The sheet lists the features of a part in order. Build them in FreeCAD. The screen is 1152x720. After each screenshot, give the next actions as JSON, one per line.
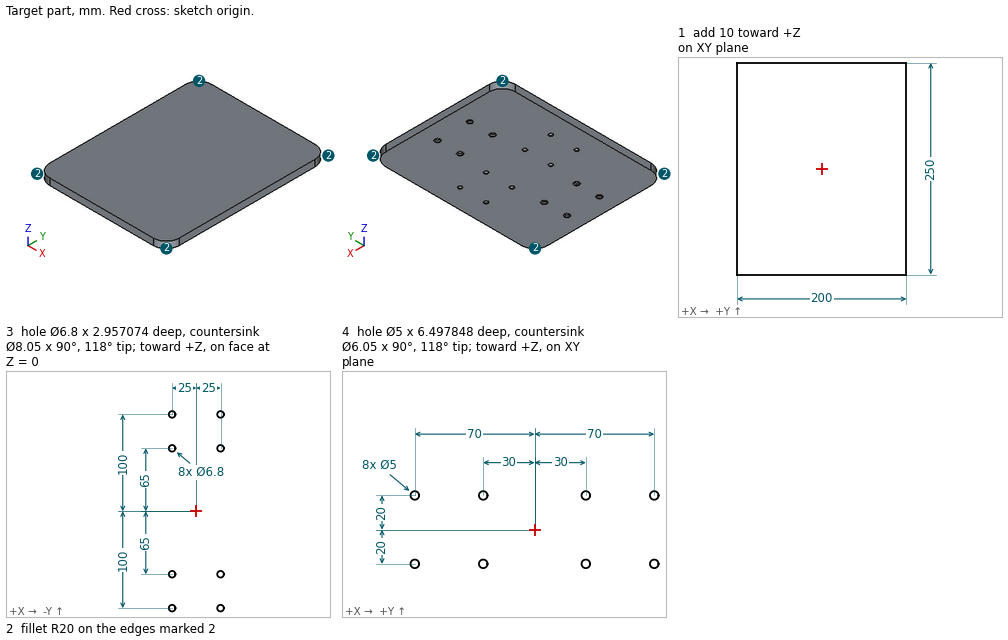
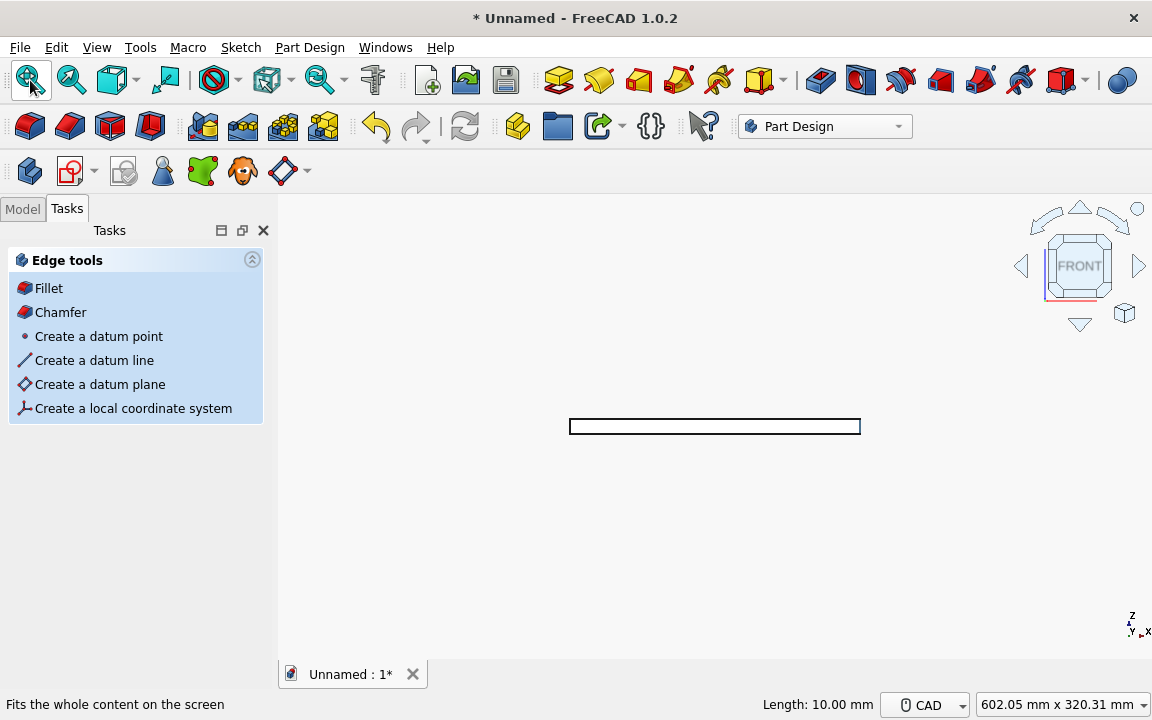
{"action": "left_click", "coordinate": [570, 426], "text": "ctrl"}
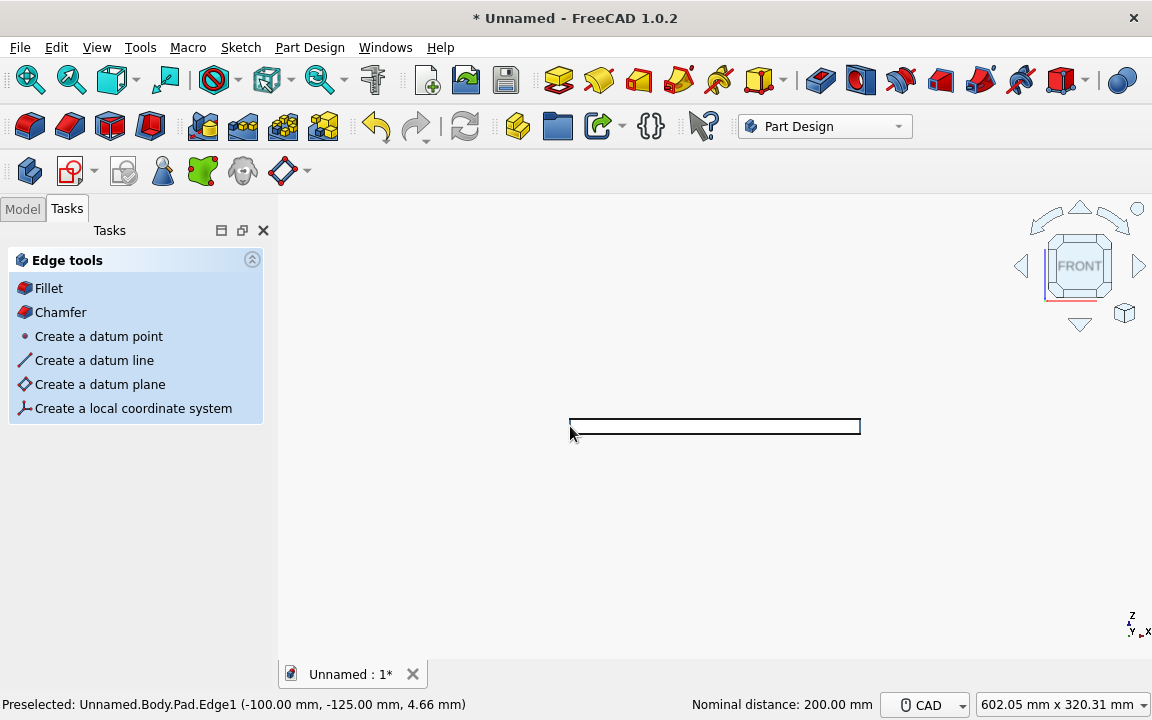
{"action": "scroll", "coordinate": [570, 426], "scroll_direction": "up", "scroll_amount": 6}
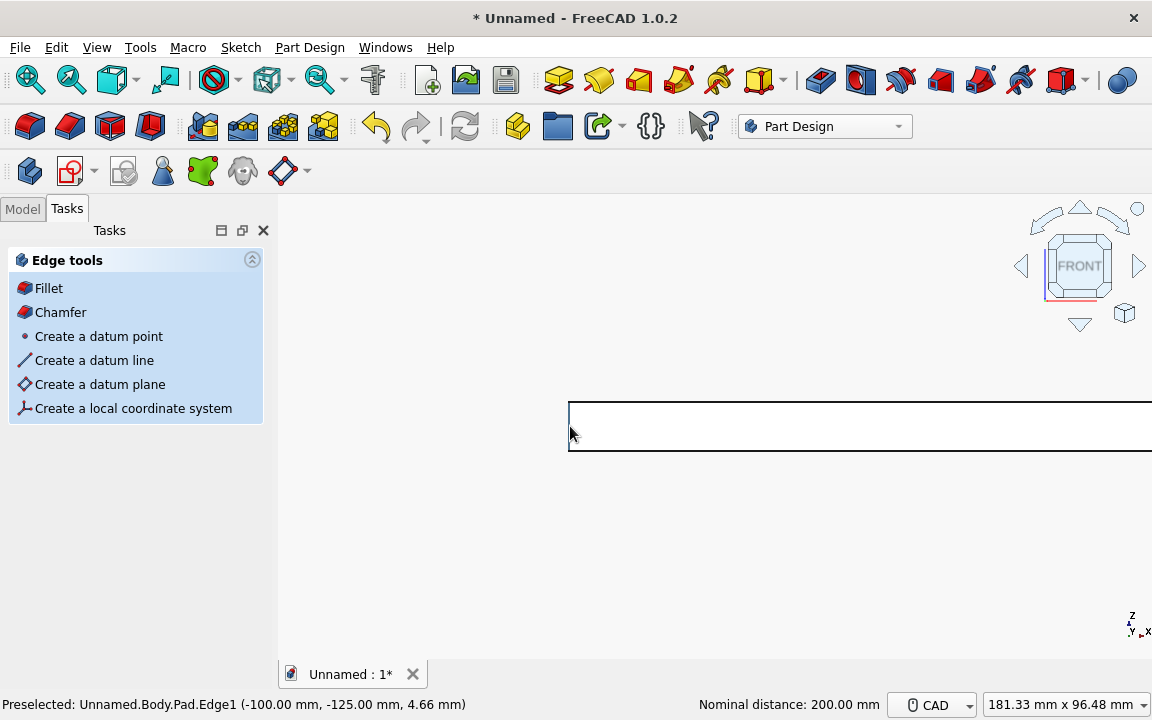
{"action": "key", "text": "v f"}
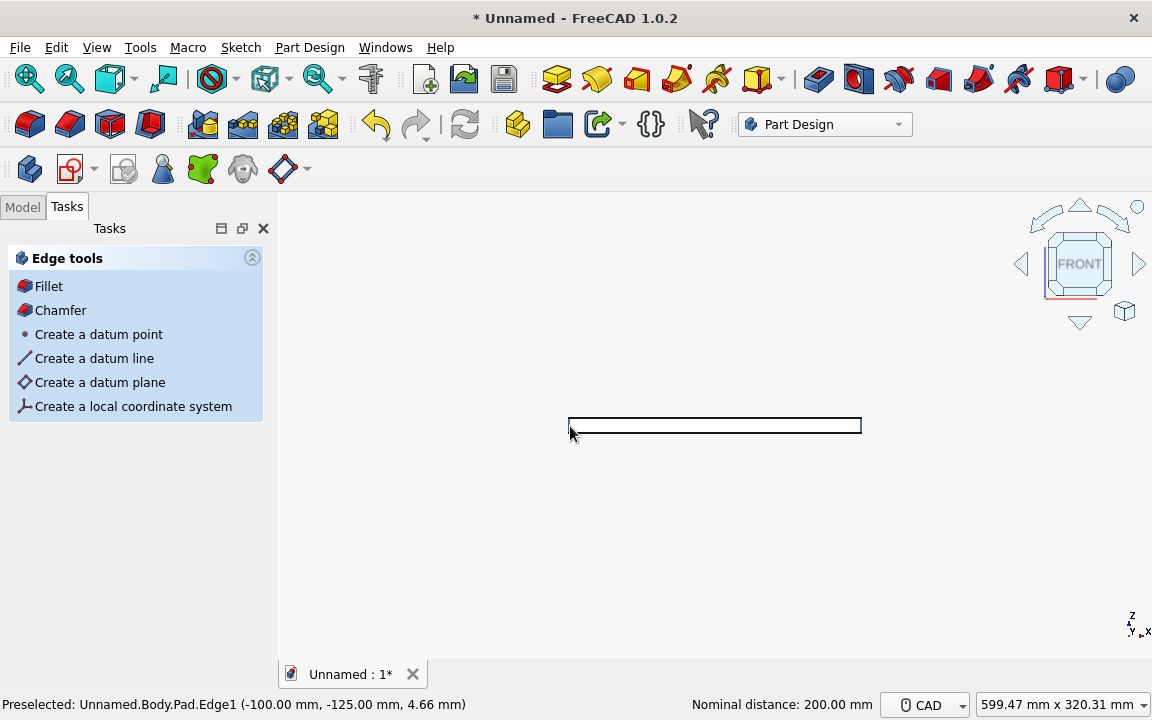
{"action": "key", "text": "3"}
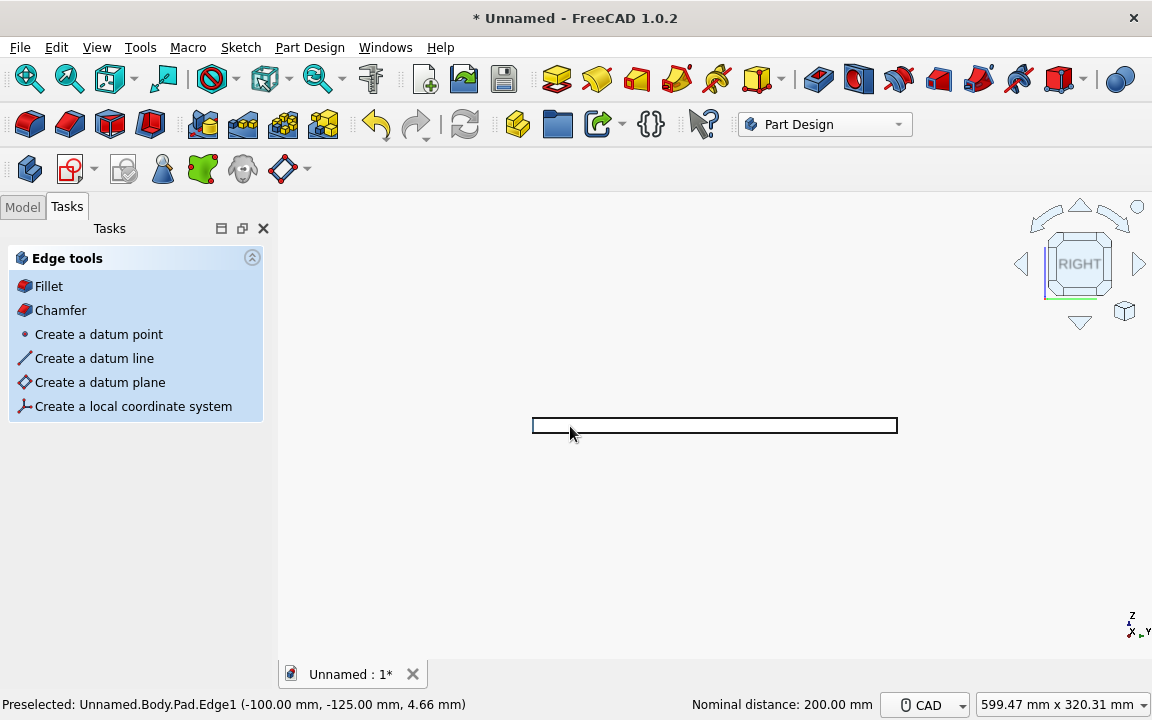
{"action": "key", "text": "v f"}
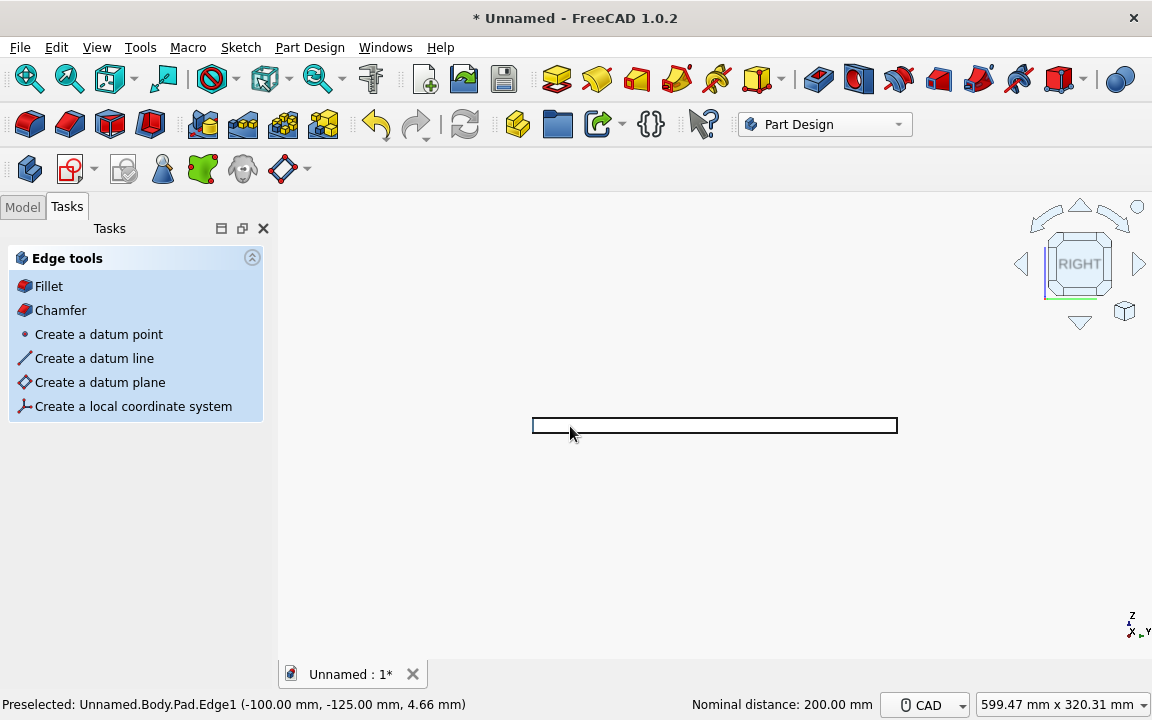
{"action": "left_click", "coordinate": [897, 424], "text": "ctrl"}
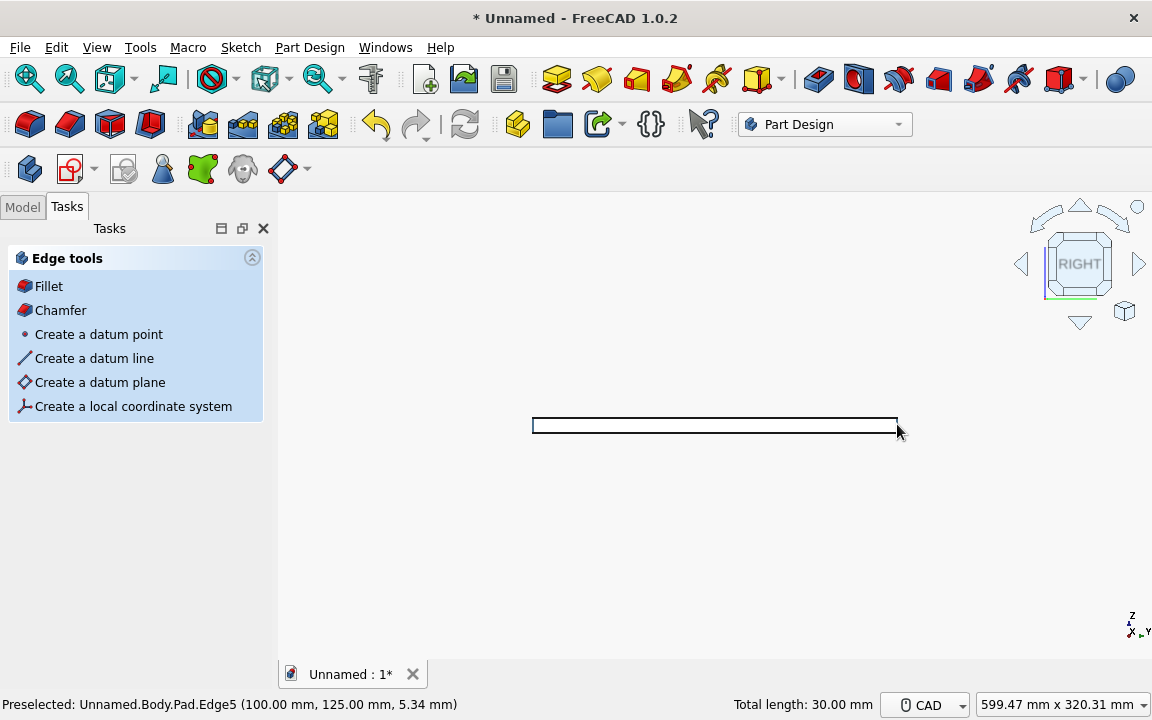
{"action": "scroll", "coordinate": [897, 424], "scroll_direction": "up", "scroll_amount": 6}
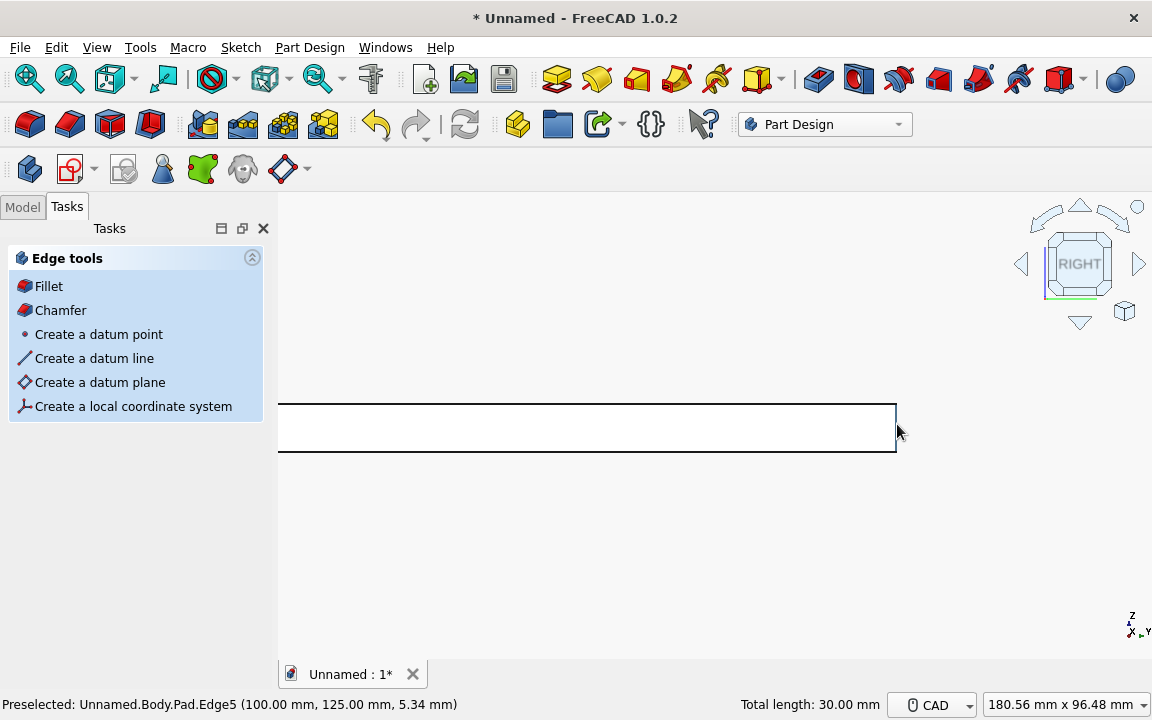
{"action": "key", "text": "v f"}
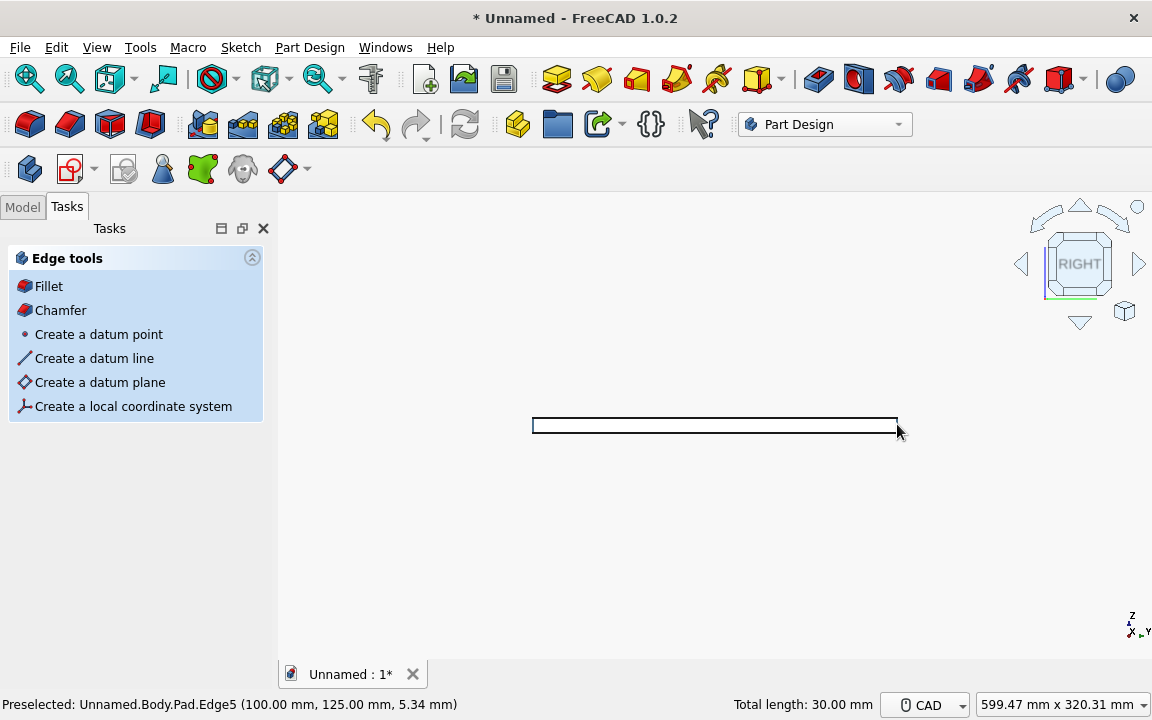
{"action": "key", "text": "5"}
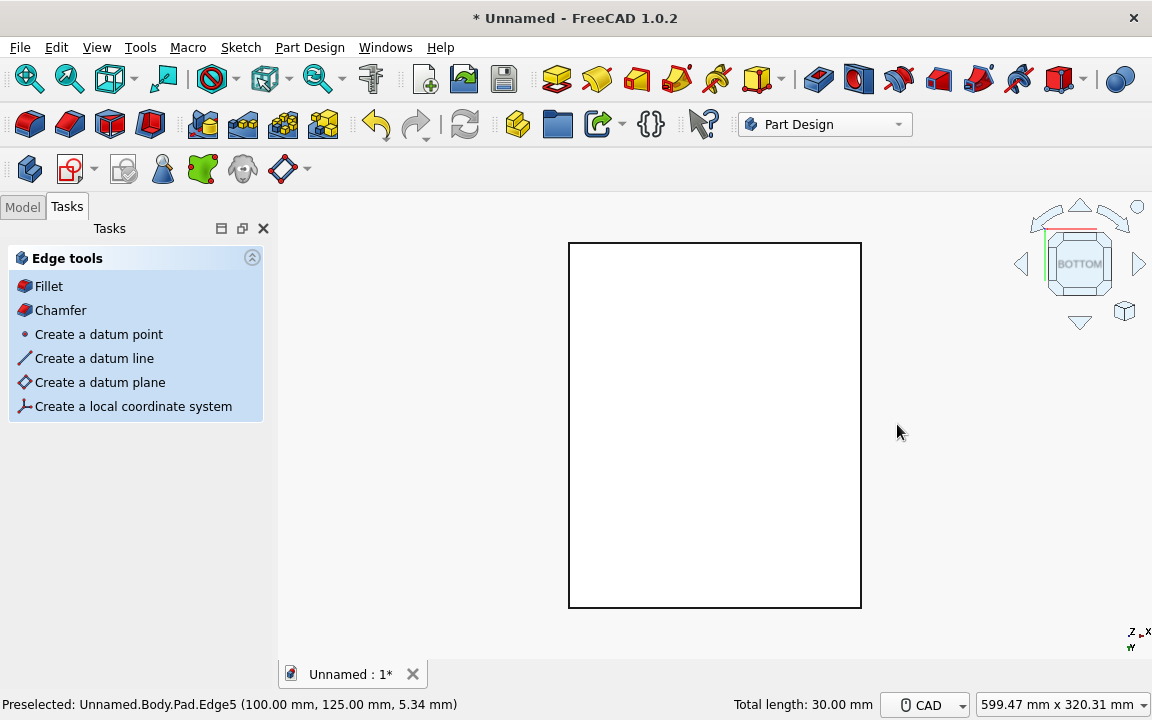
{"action": "scroll", "coordinate": [569, 607], "scroll_direction": "up", "scroll_amount": 6}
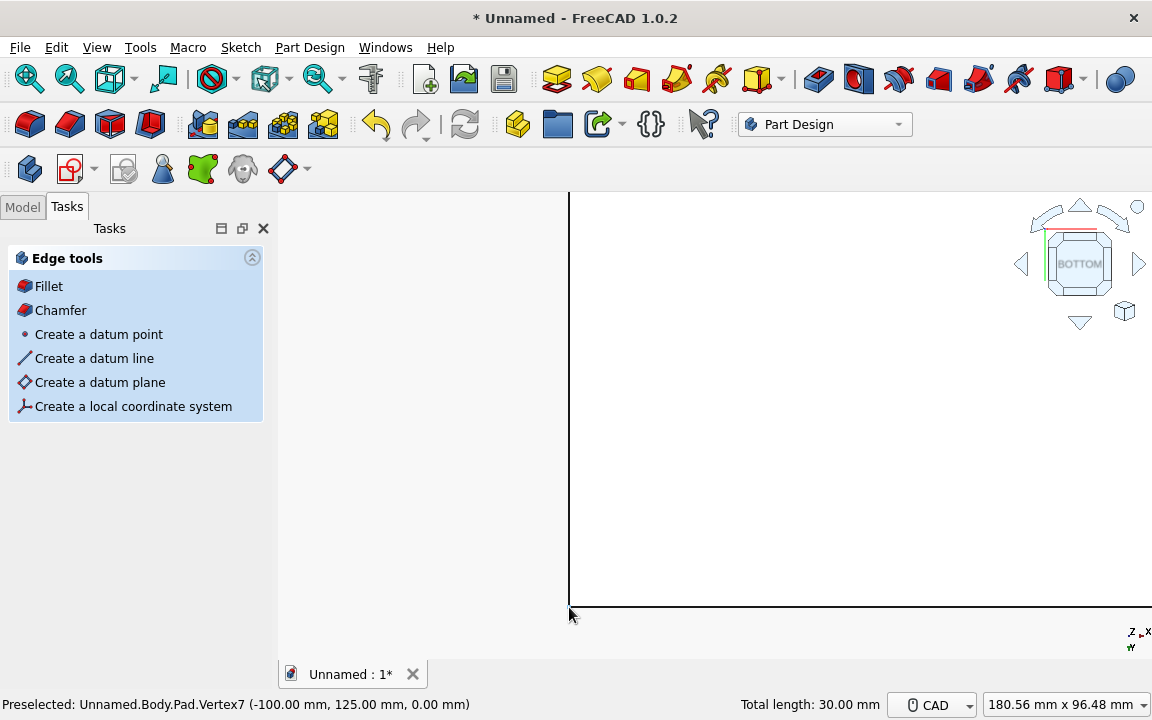
{"action": "key", "text": "v f"}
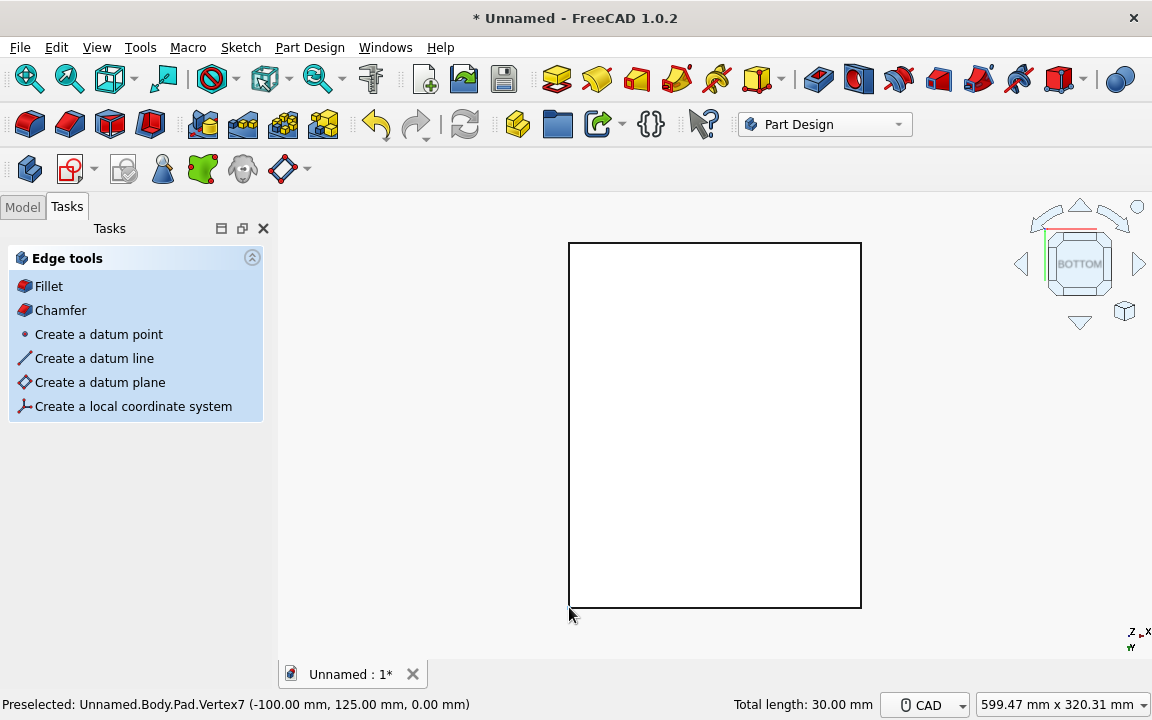
{"action": "key", "text": "4"}